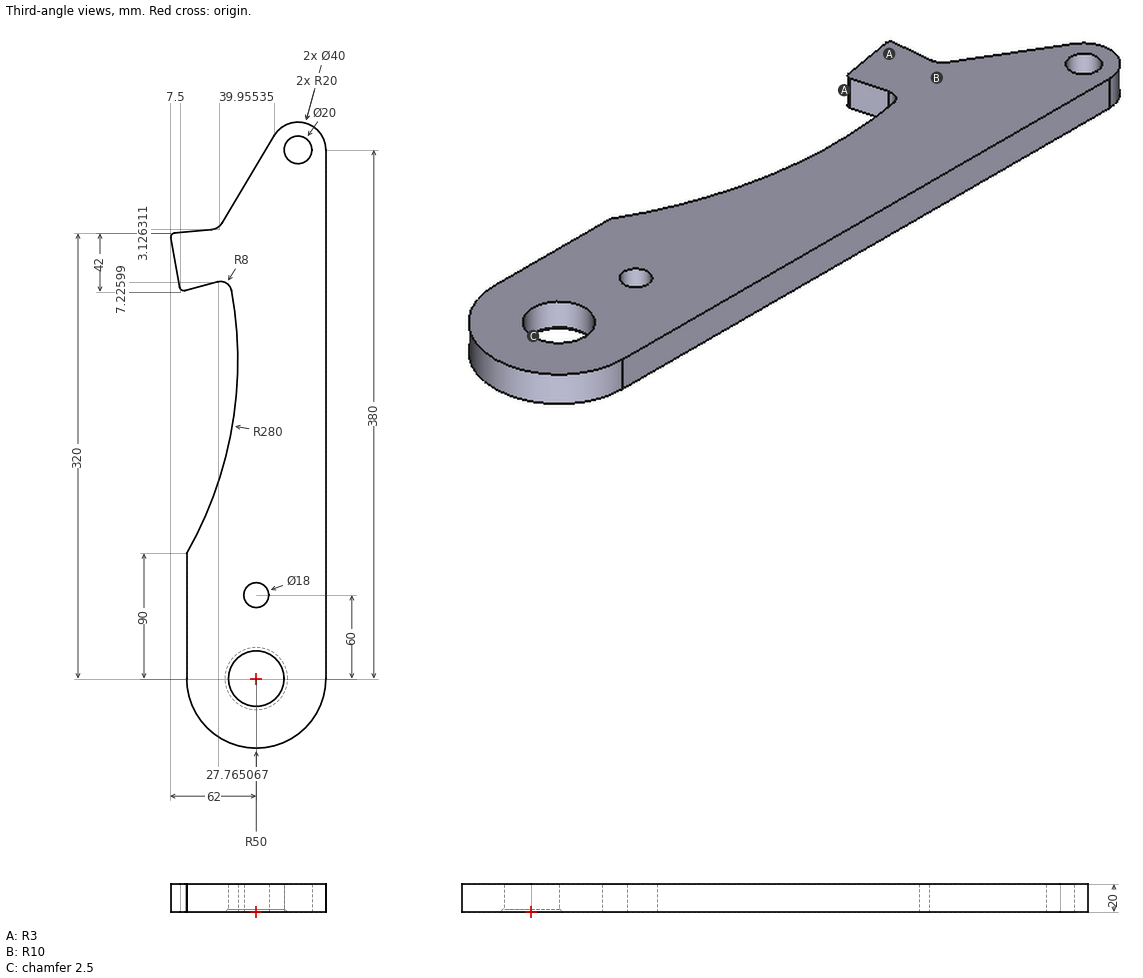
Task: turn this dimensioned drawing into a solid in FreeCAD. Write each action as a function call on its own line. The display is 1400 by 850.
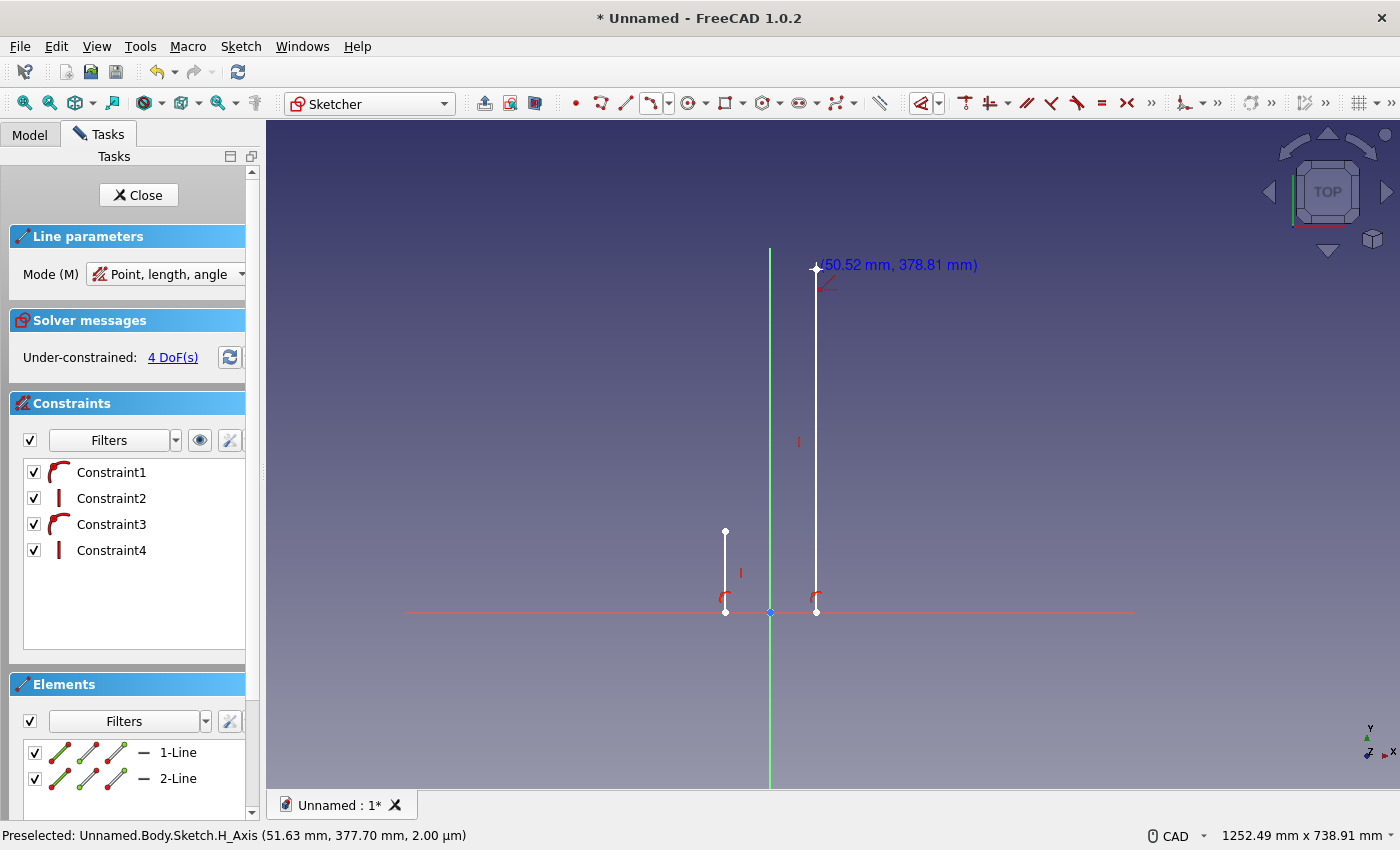
click(601, 104)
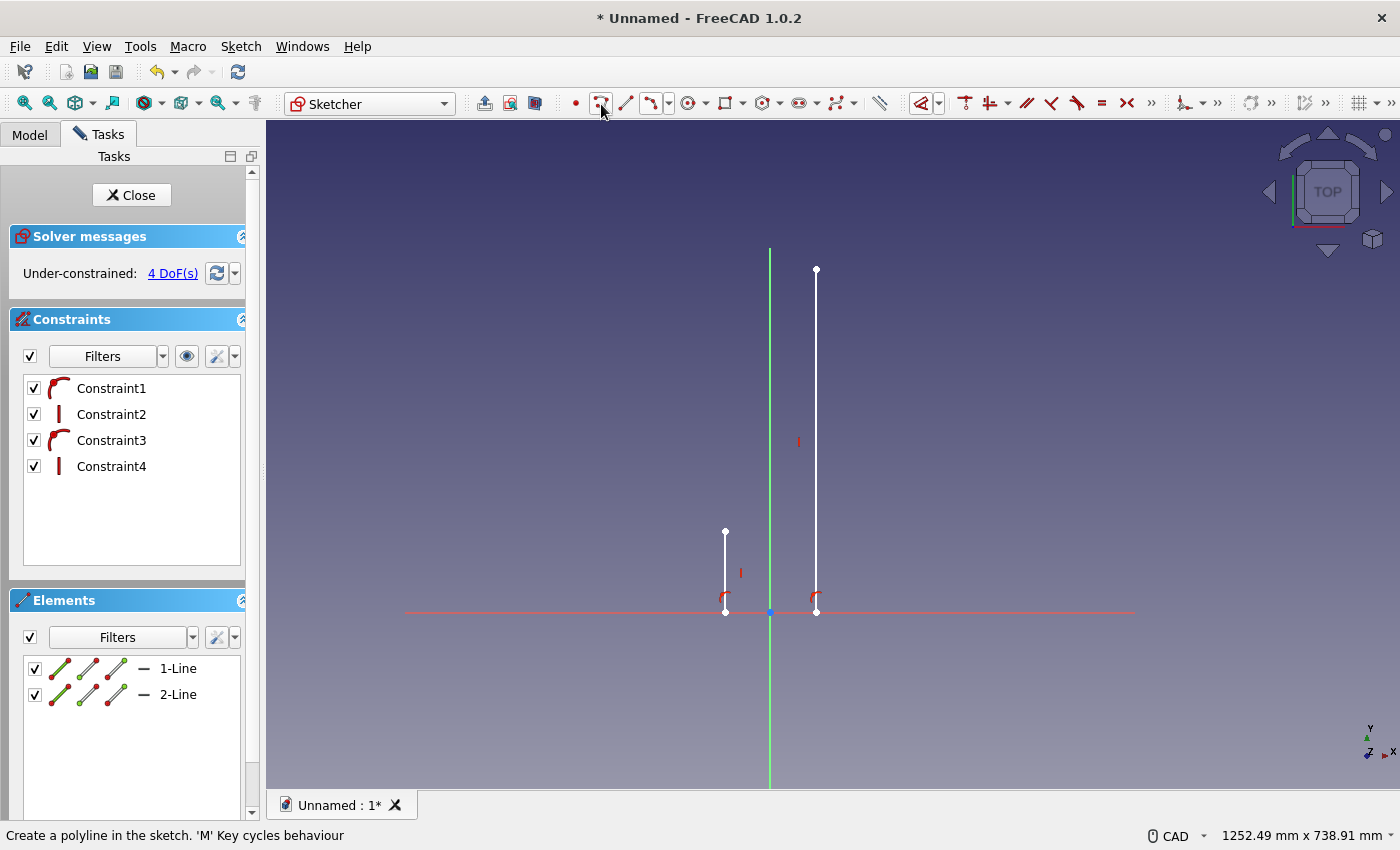
scroll(782, 260, up, 2)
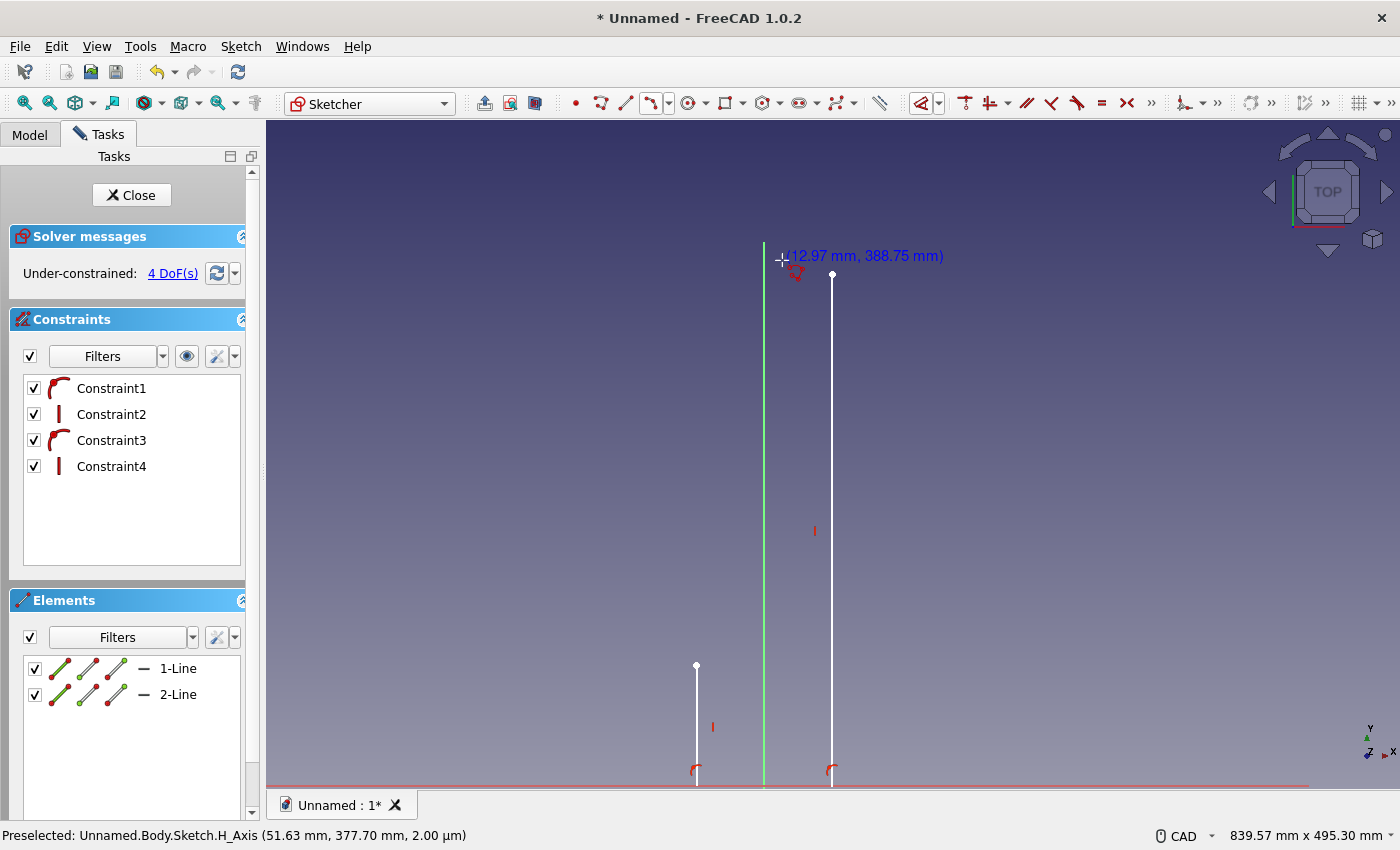
click(782, 259)
click(728, 350)
click(681, 354)
click(691, 411)
click(727, 401)
right_click(727, 401)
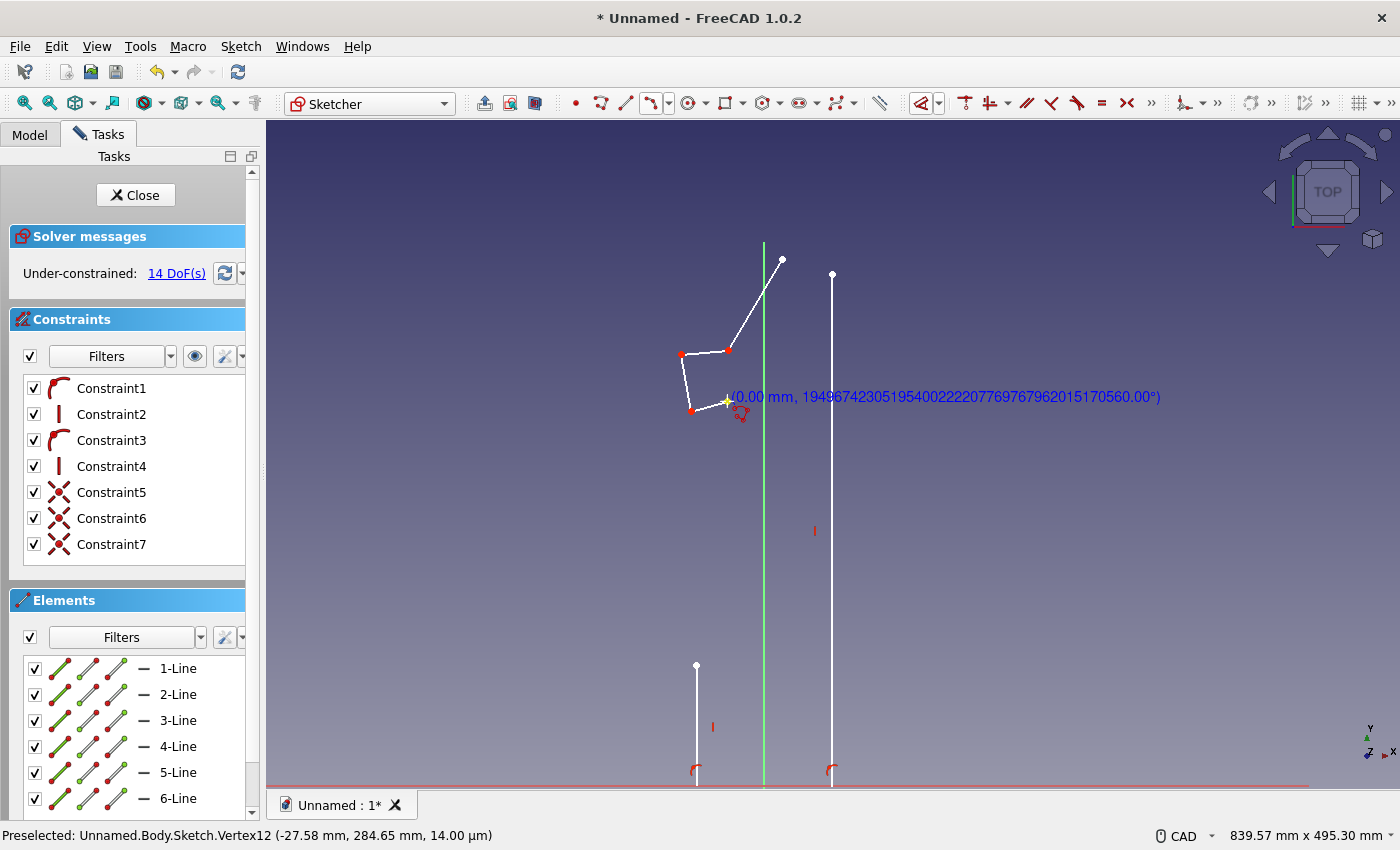
click(650, 104)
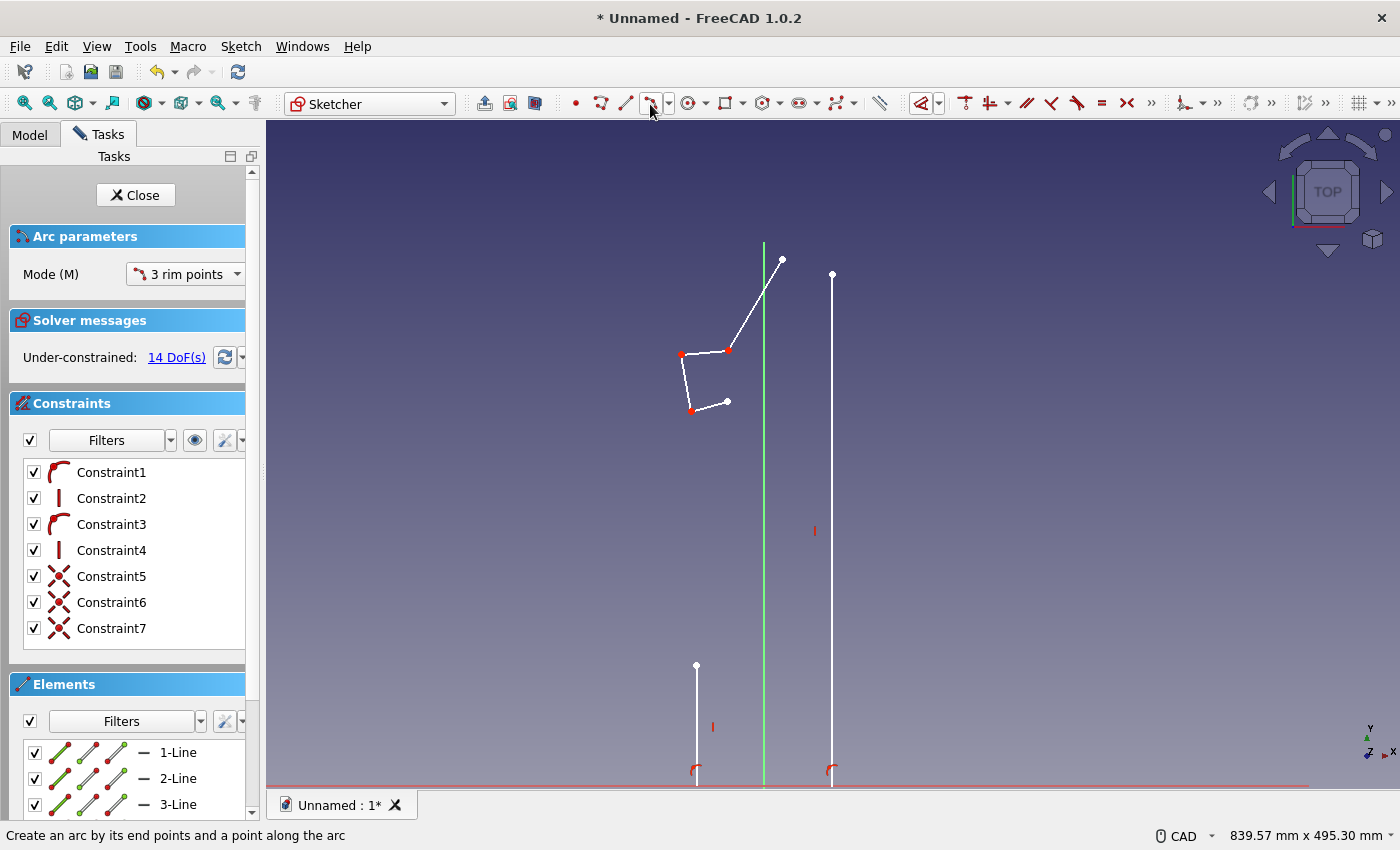
scroll(781, 259, down, 2)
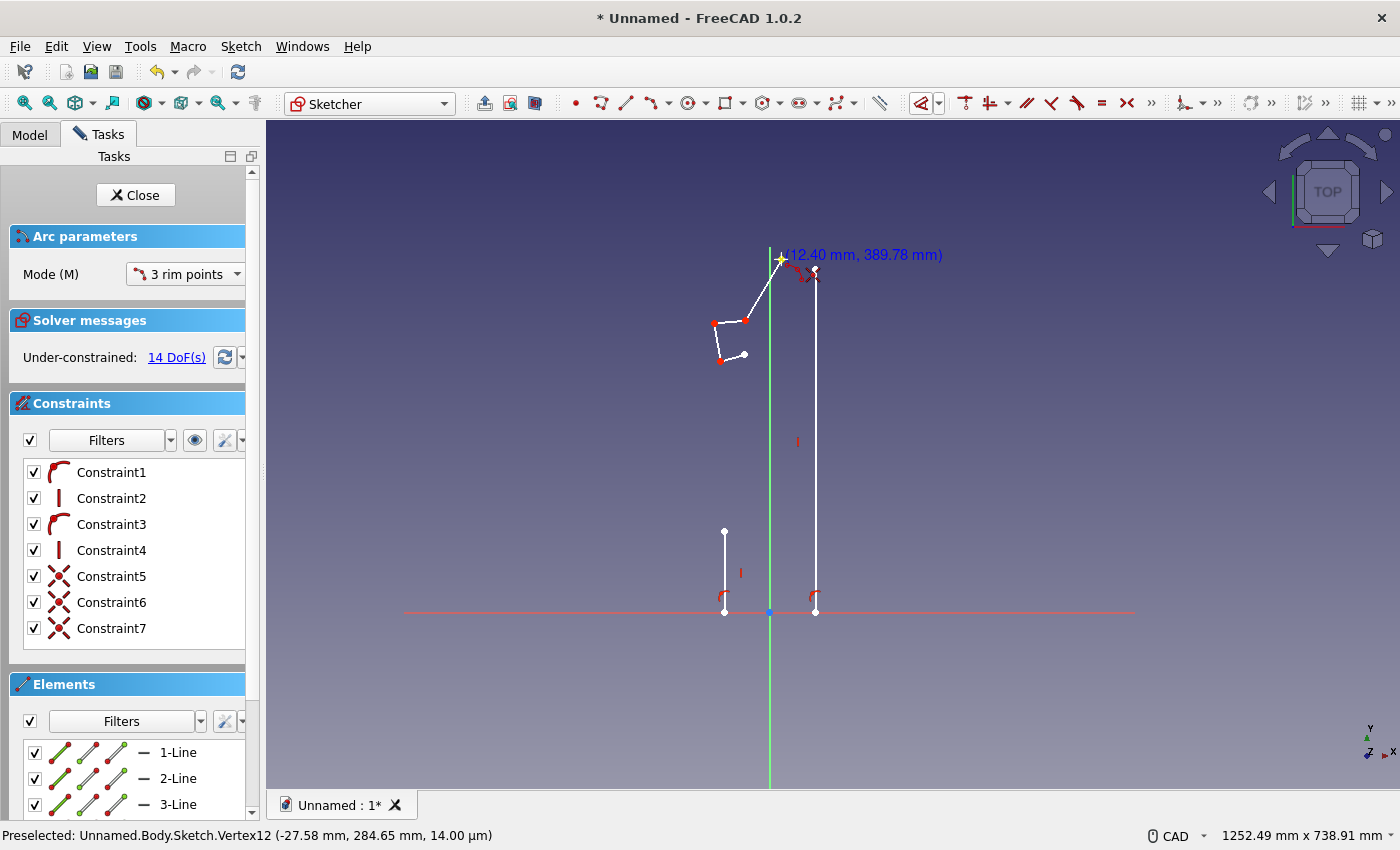
click(725, 613)
click(816, 613)
click(743, 649)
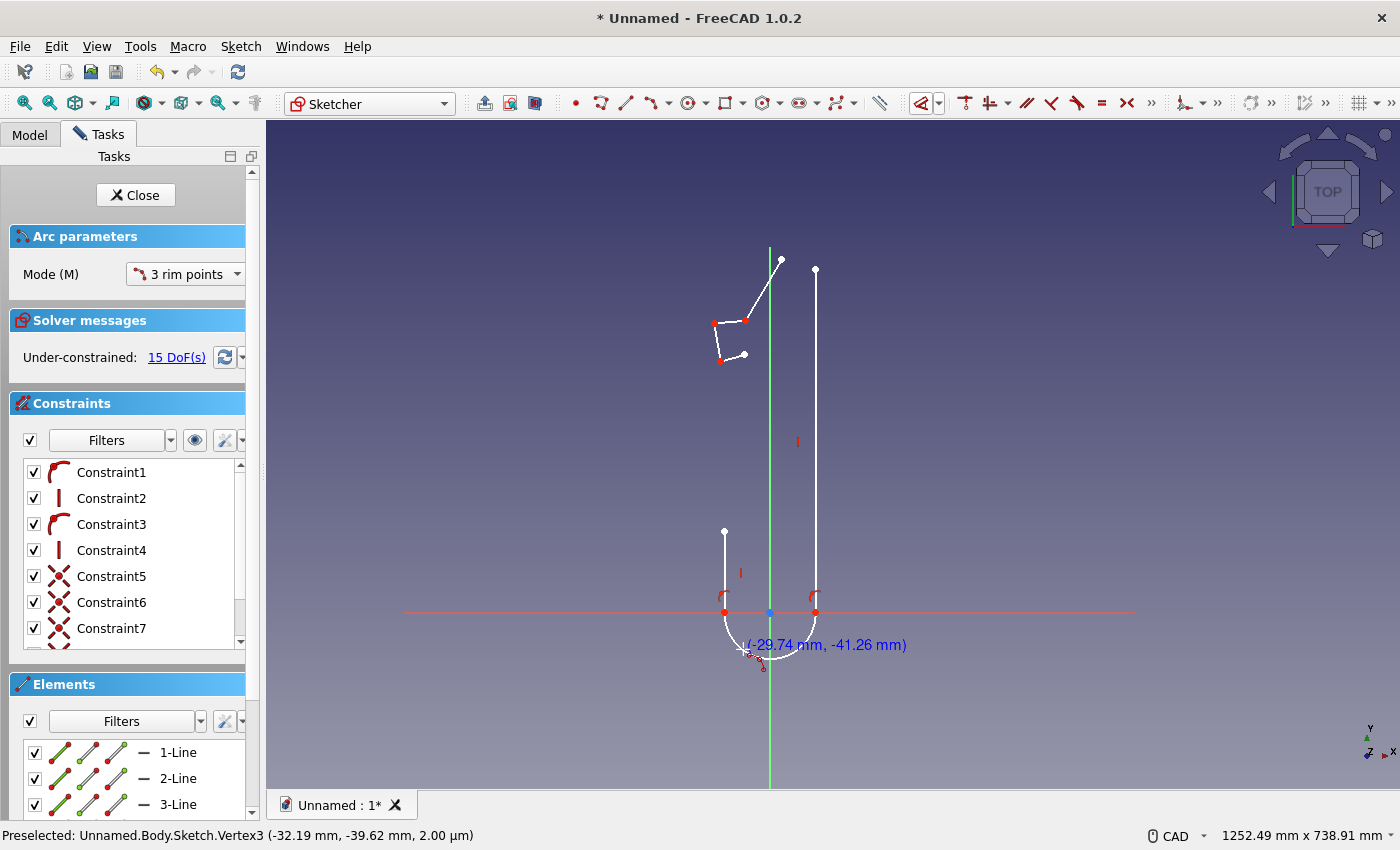
click(816, 270)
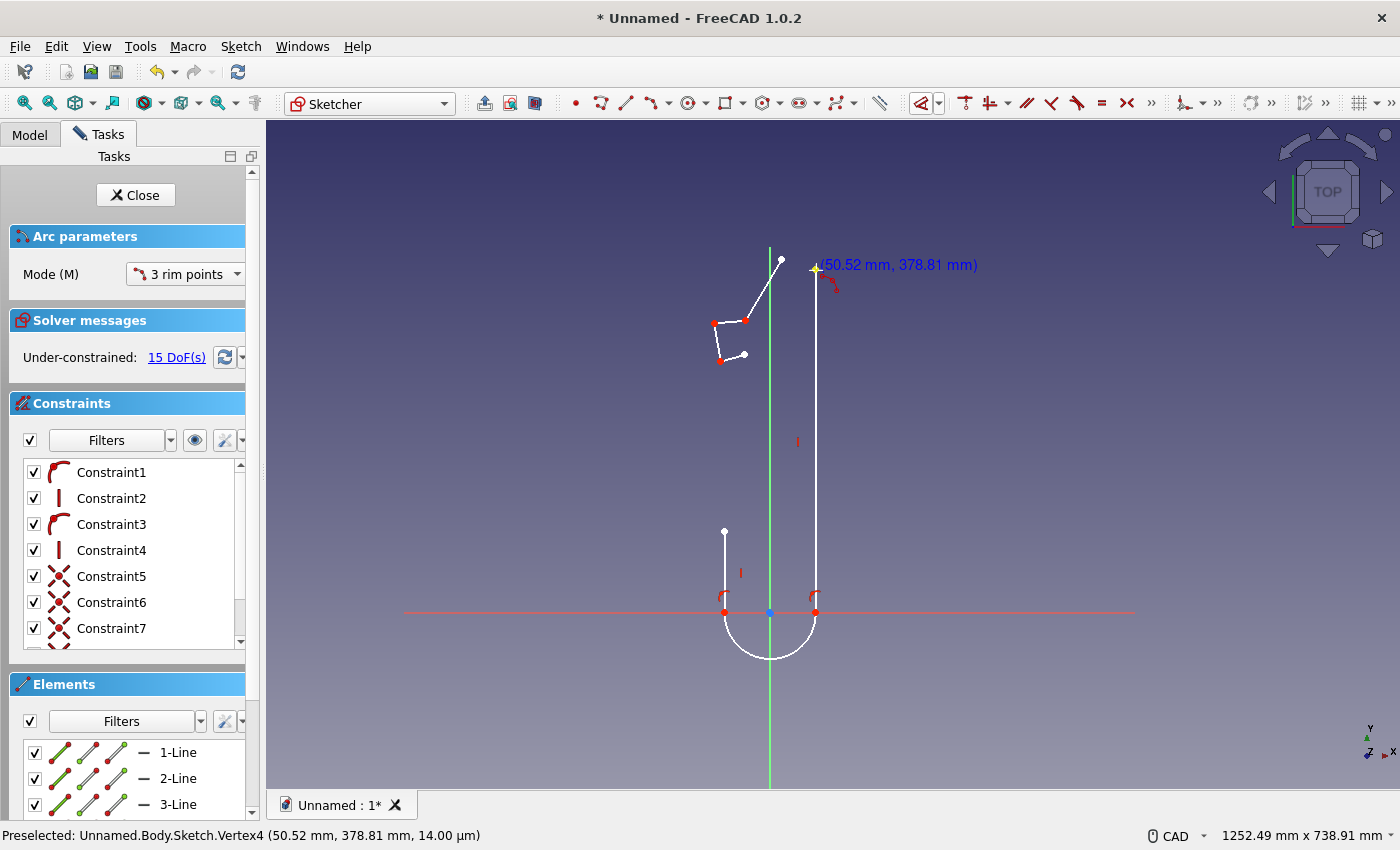
scroll(782, 259, up, 2)